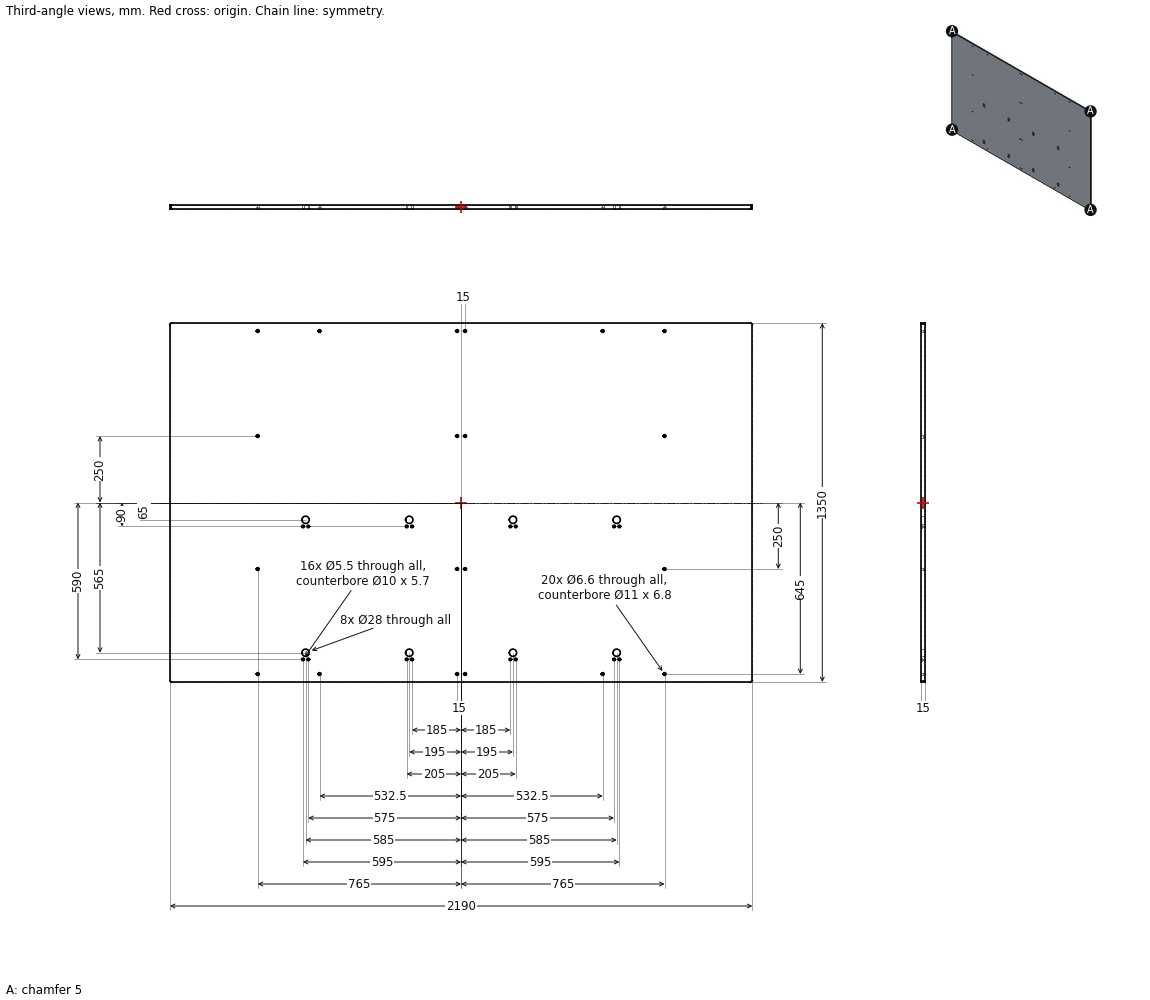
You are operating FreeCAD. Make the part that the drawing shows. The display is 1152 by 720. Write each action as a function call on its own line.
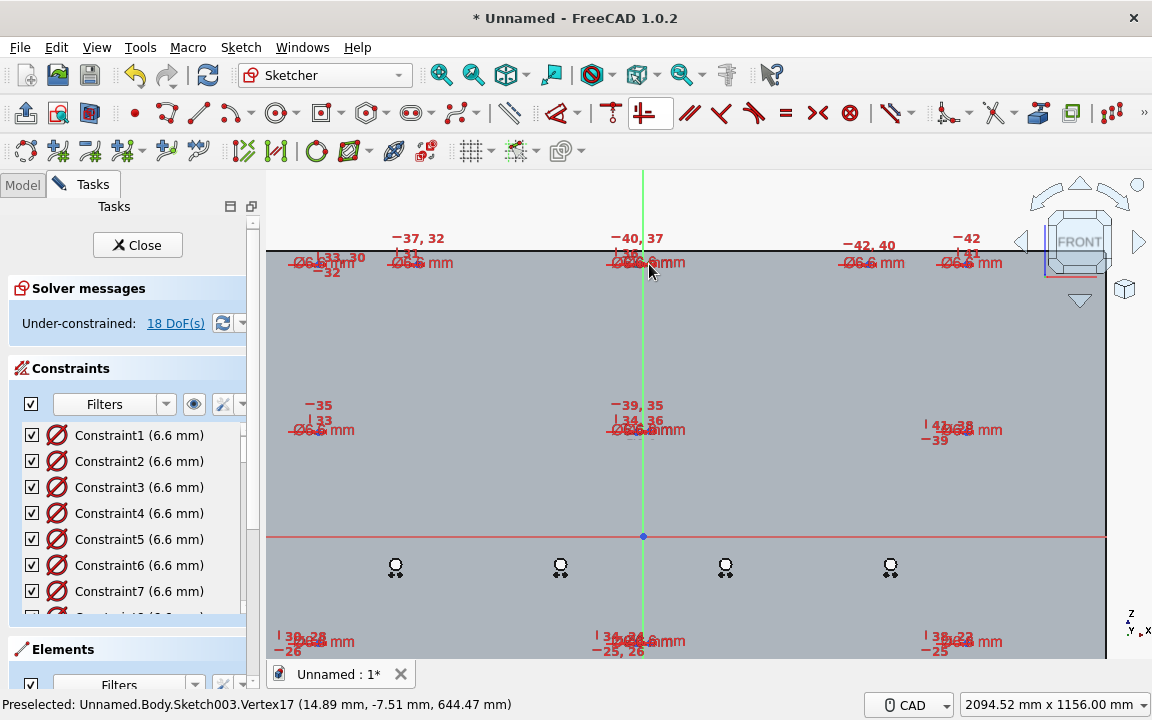
click(668, 114)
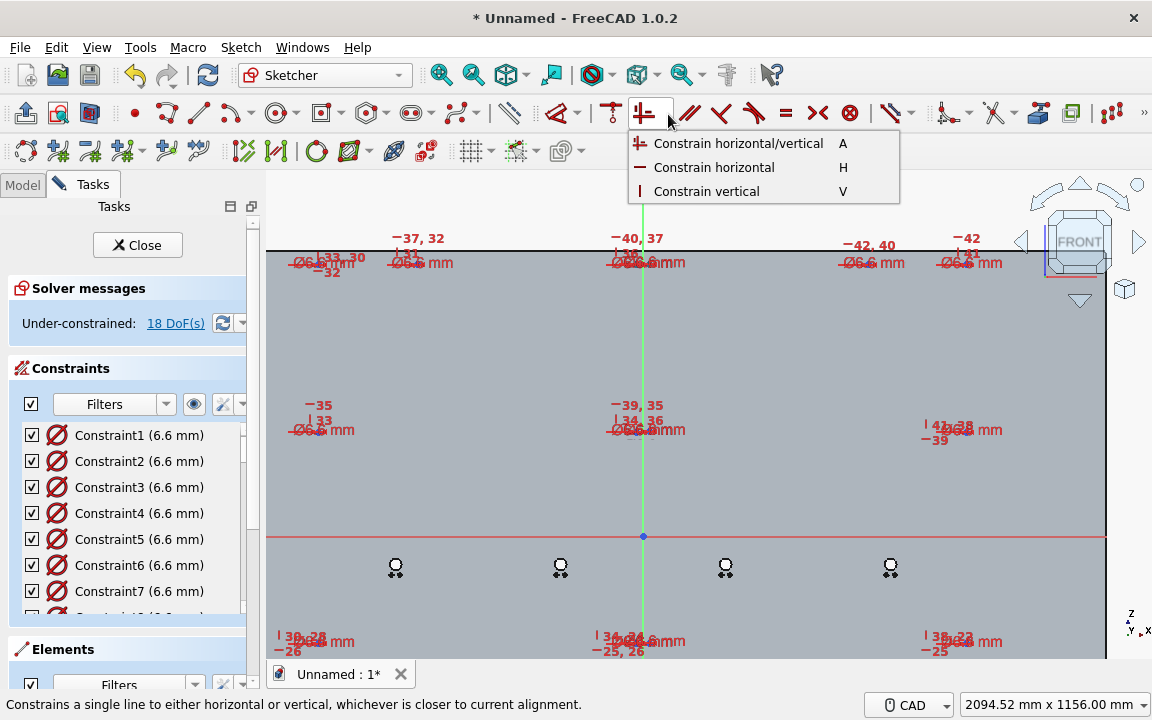
click(764, 167)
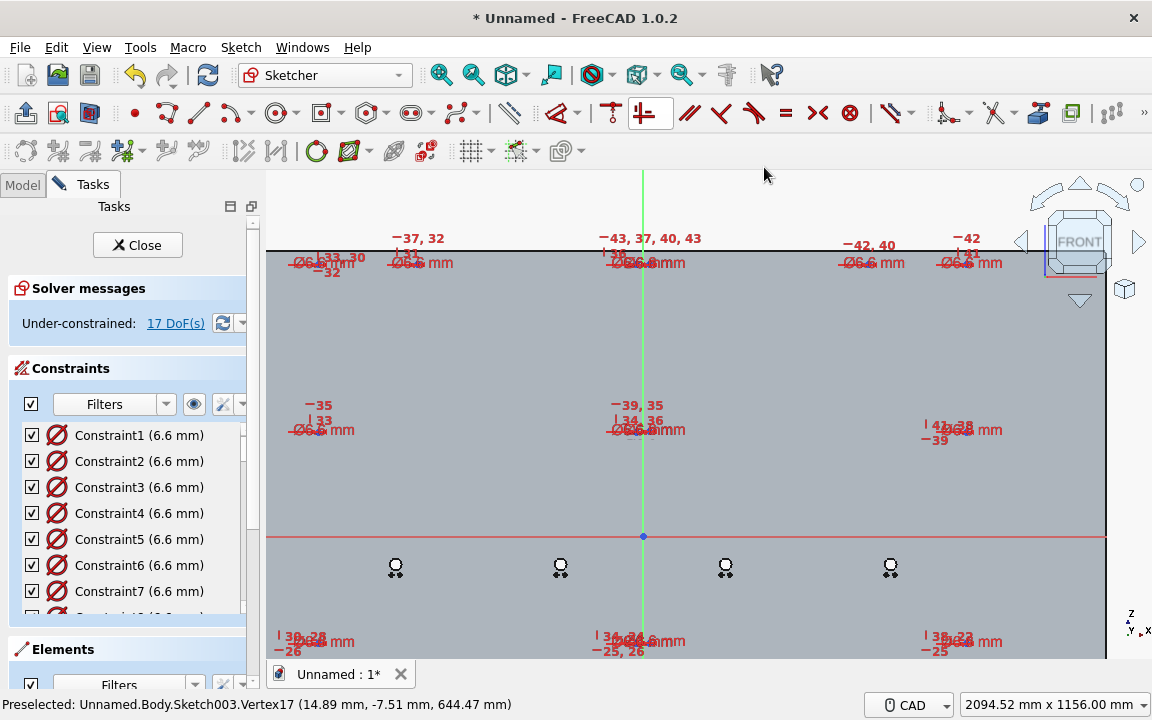
click(649, 265)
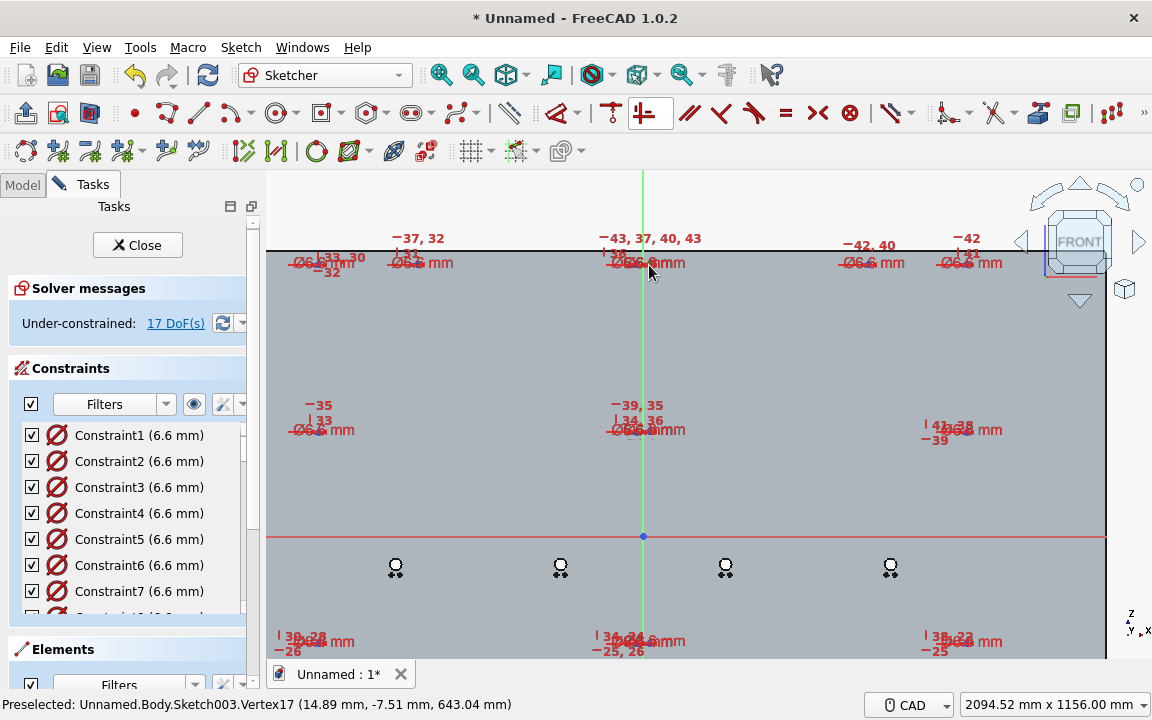
click(649, 432)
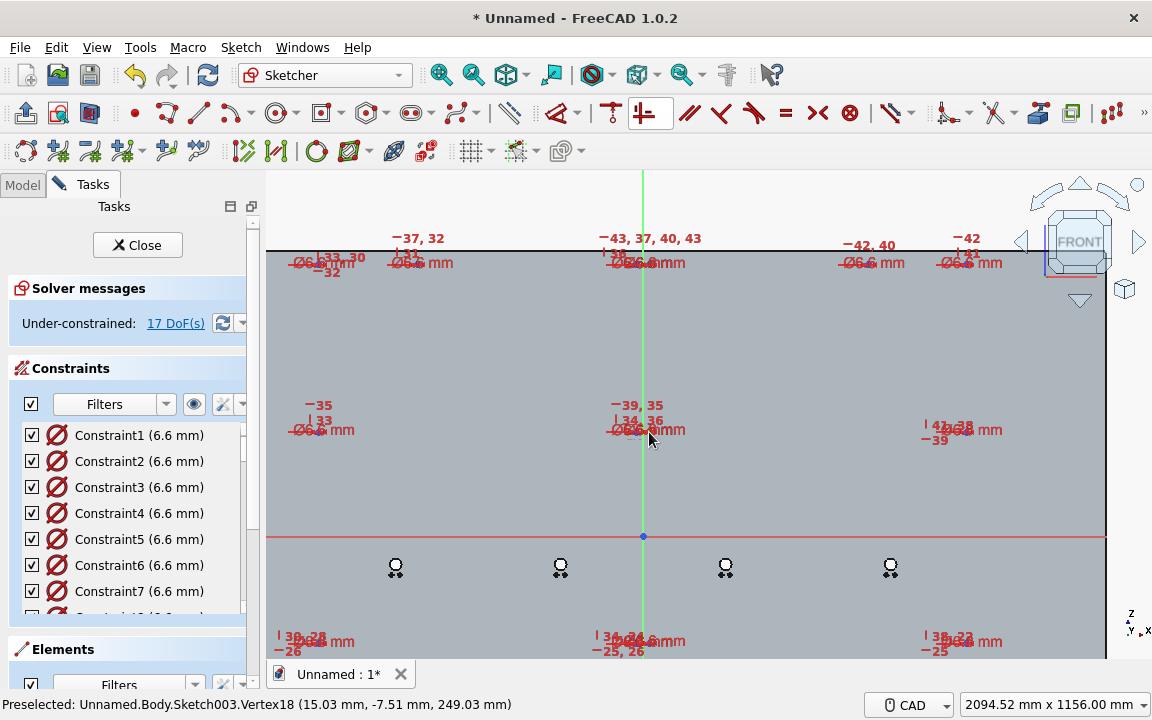
key(v)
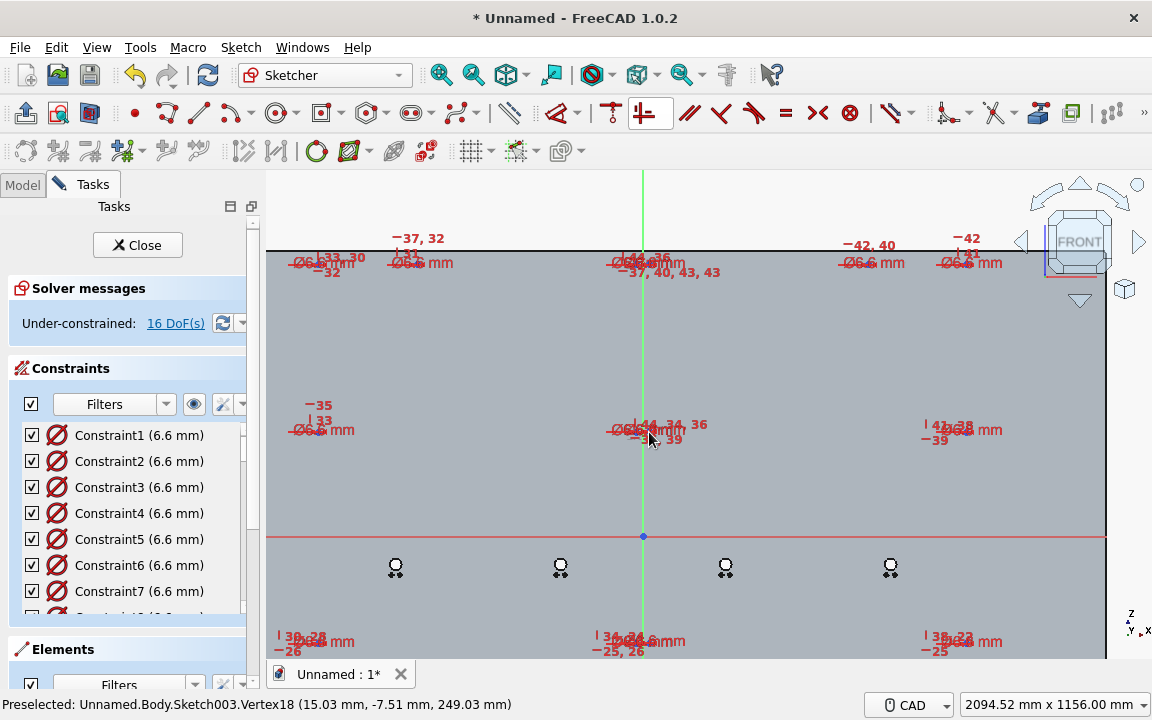
scroll(637, 432, up, 4)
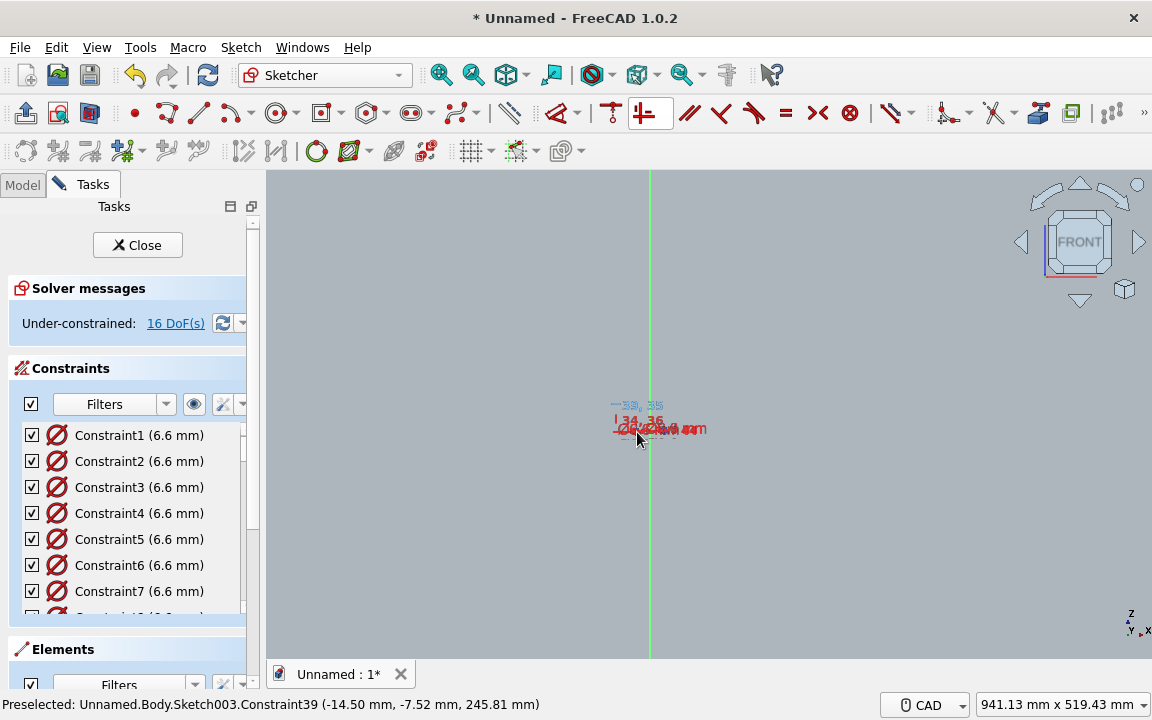
click(636, 432)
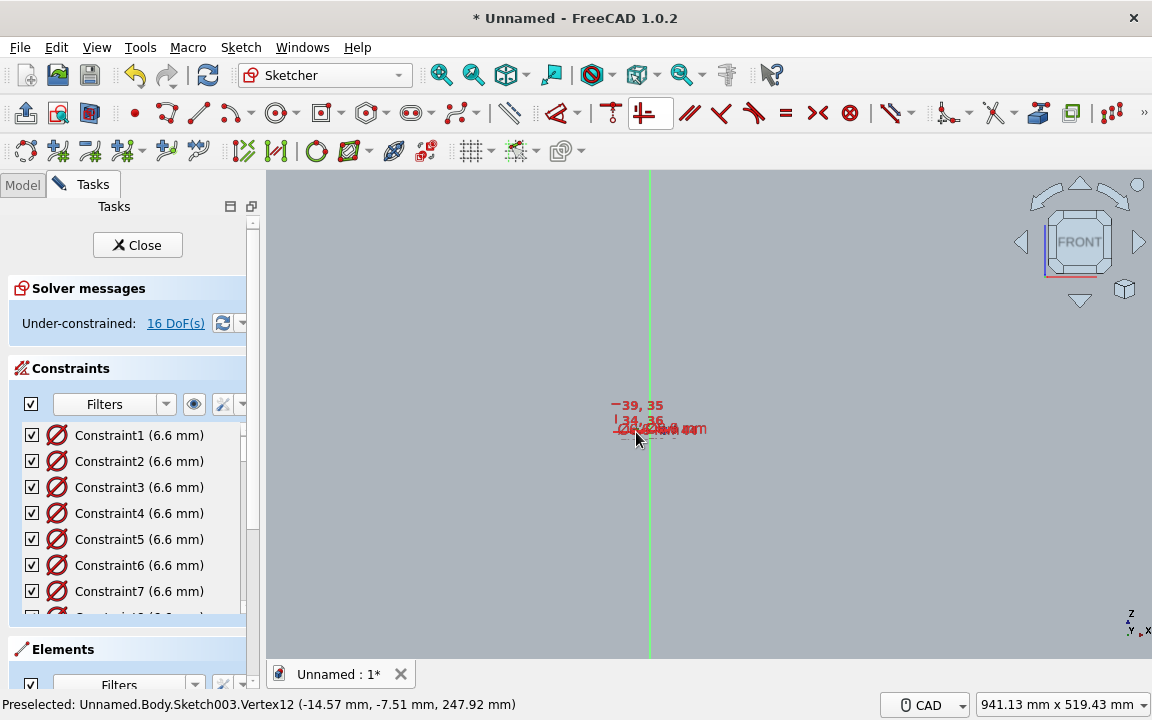
click(664, 431)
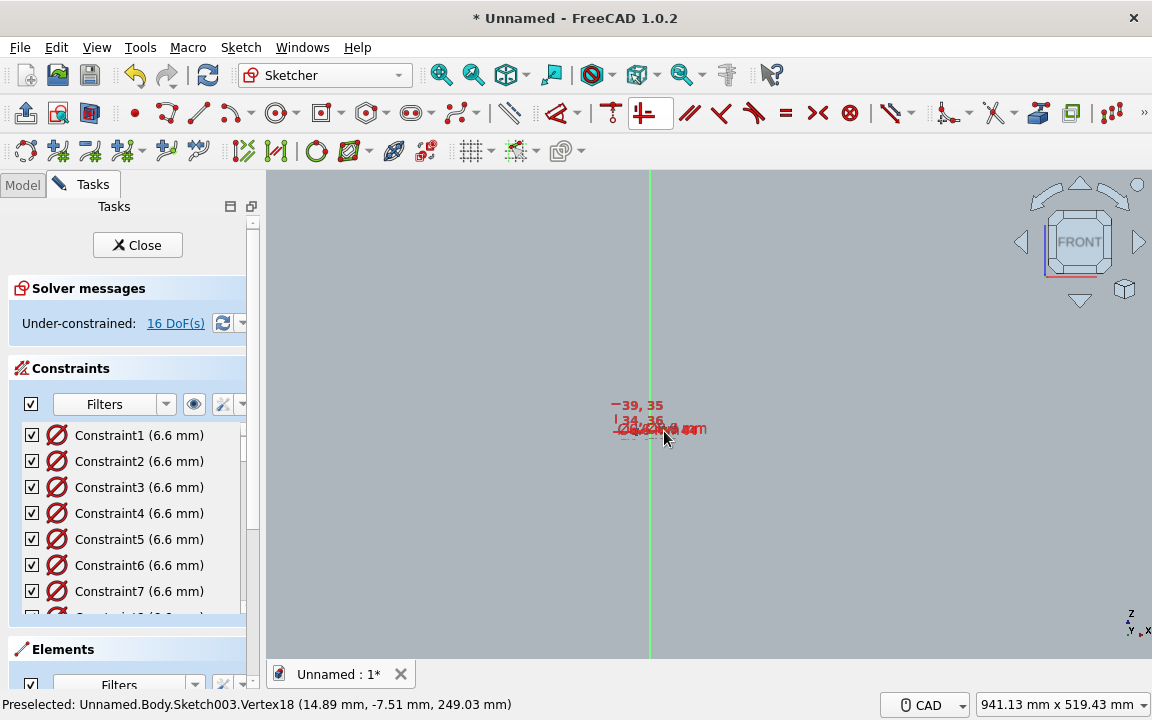
click(668, 114)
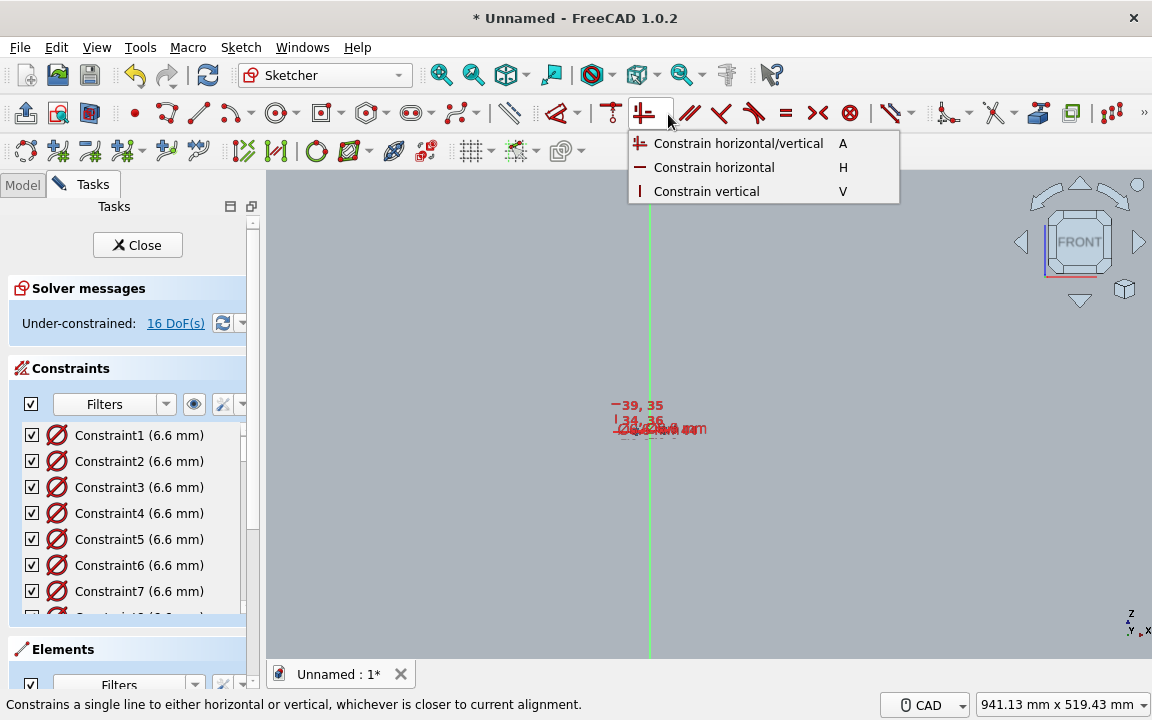
click(764, 167)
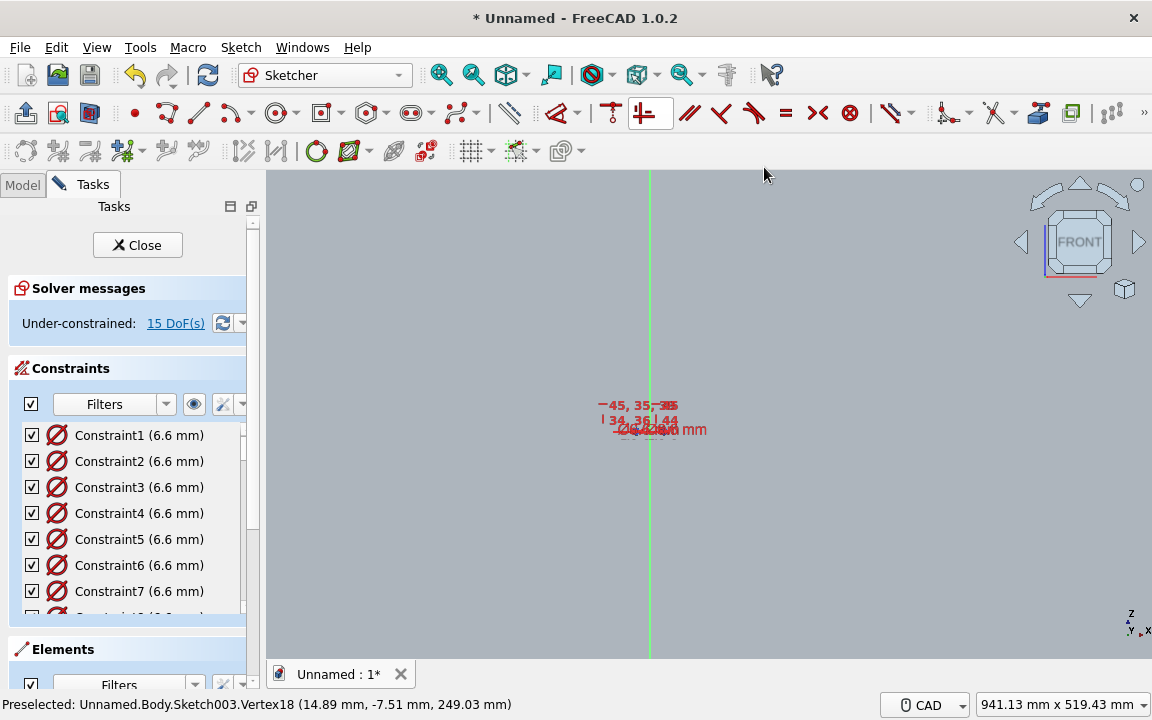
click(664, 432)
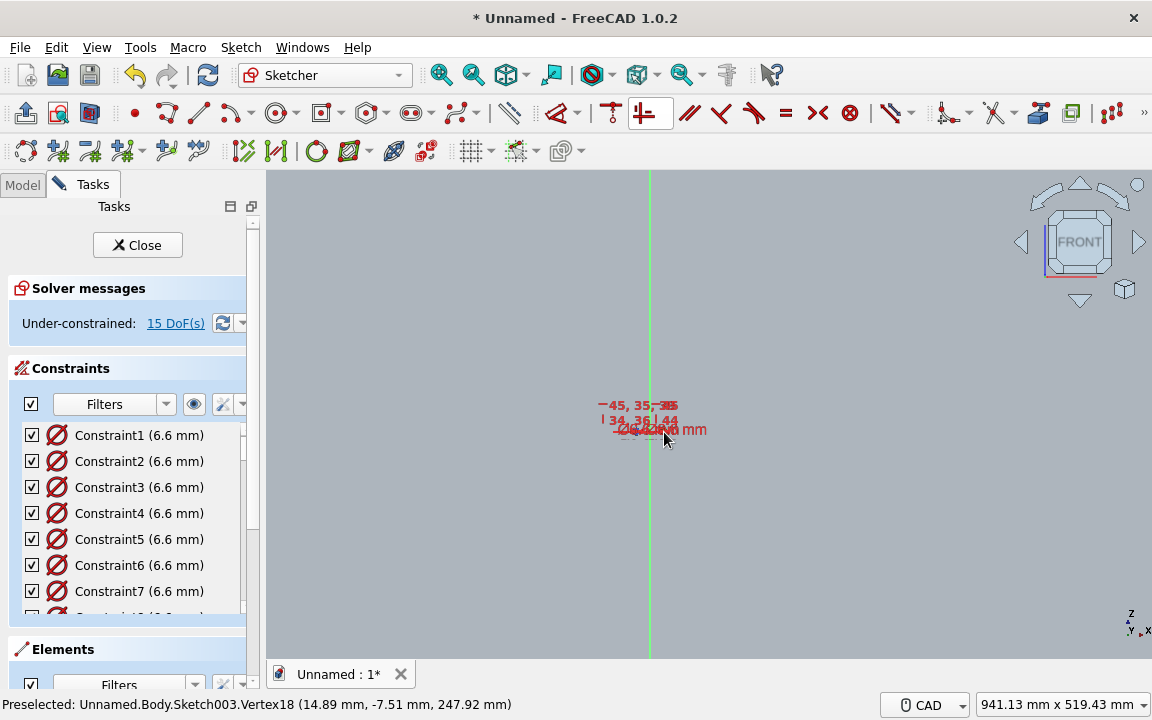
scroll(637, 333, down, 7)